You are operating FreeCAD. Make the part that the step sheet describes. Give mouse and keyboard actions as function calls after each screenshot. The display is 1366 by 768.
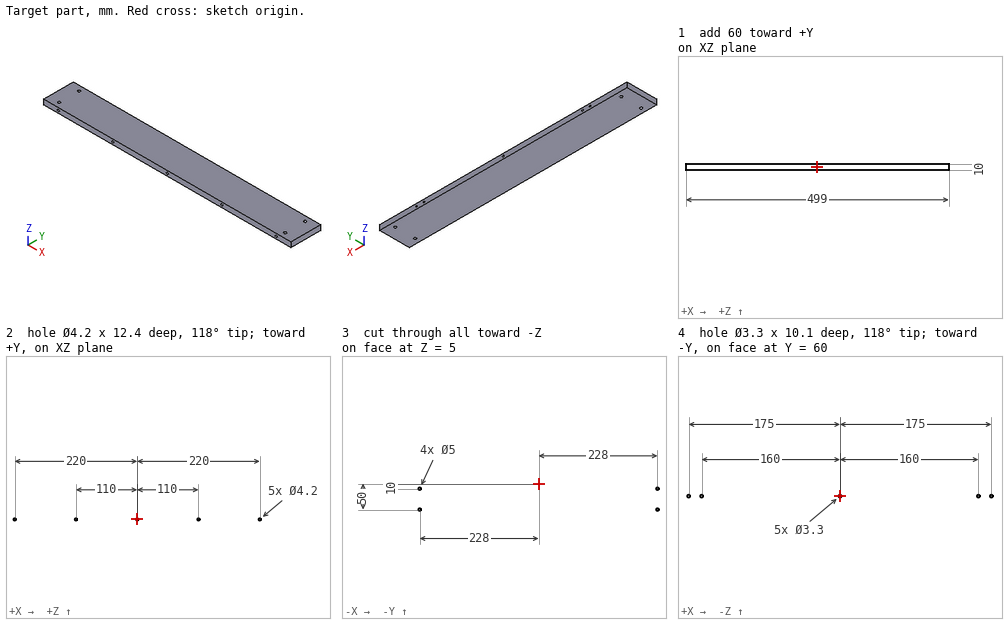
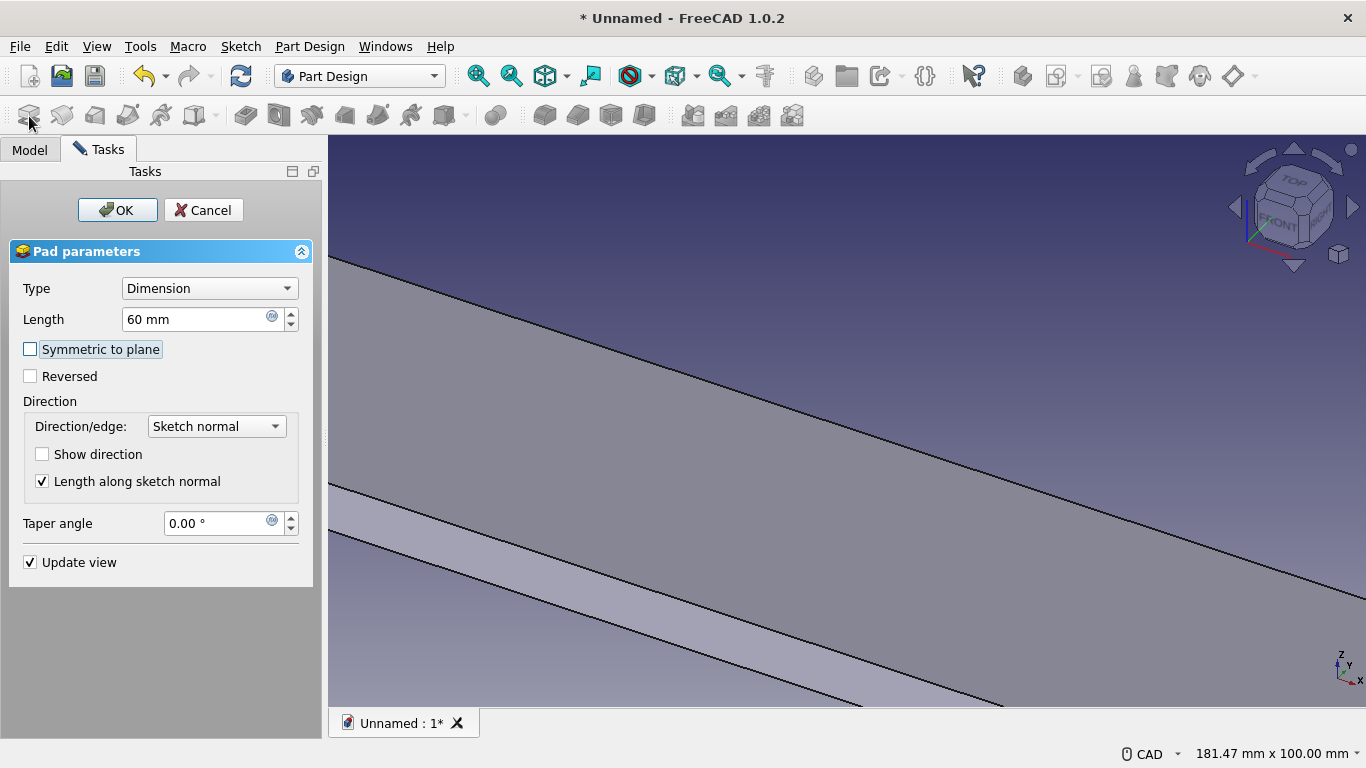
click(31, 376)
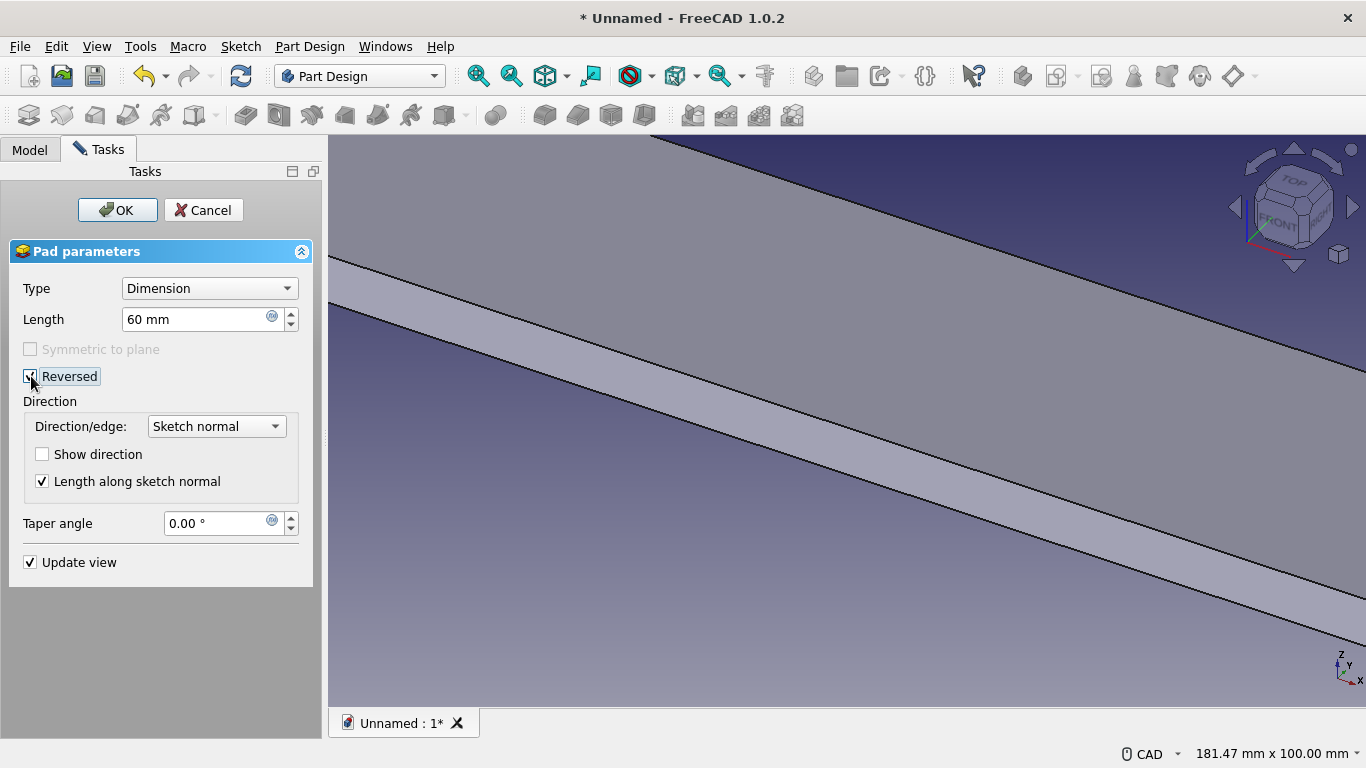
click(118, 210)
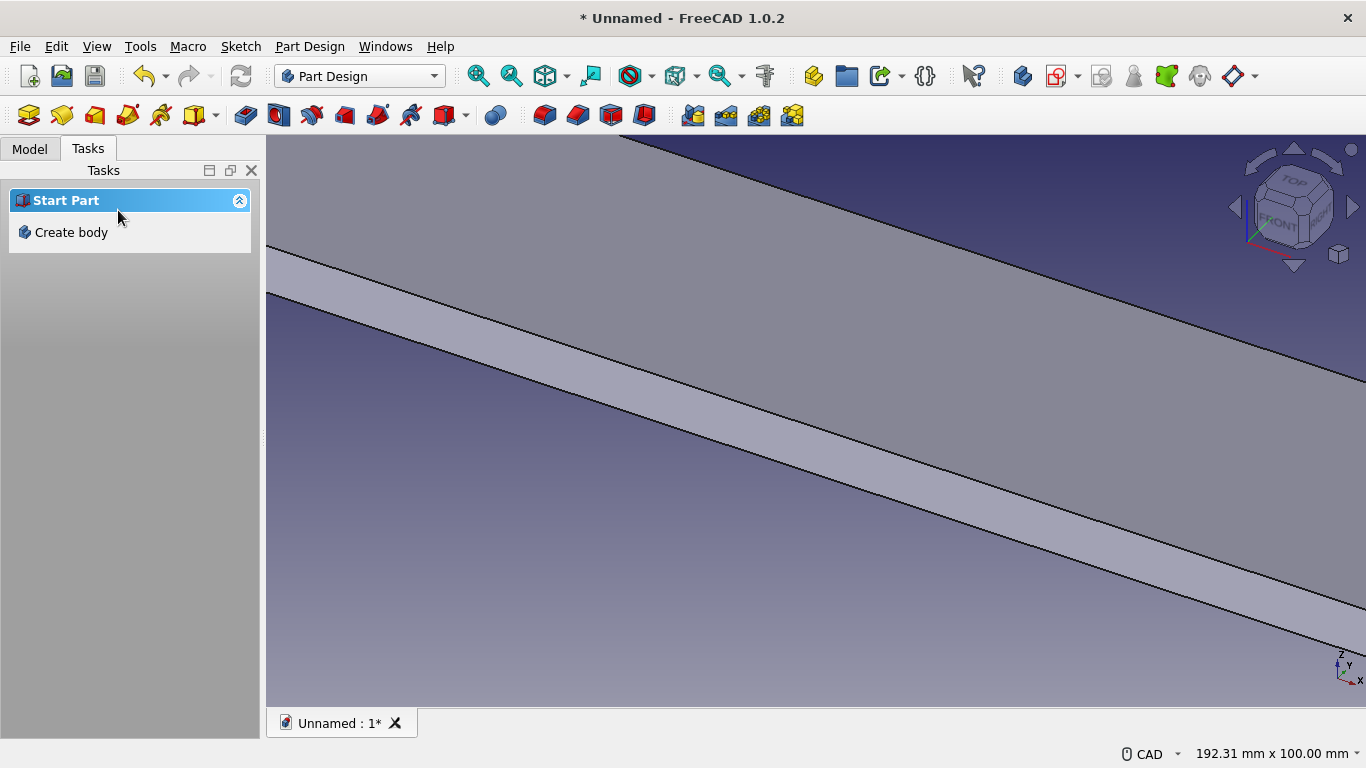
key(v)
key(f)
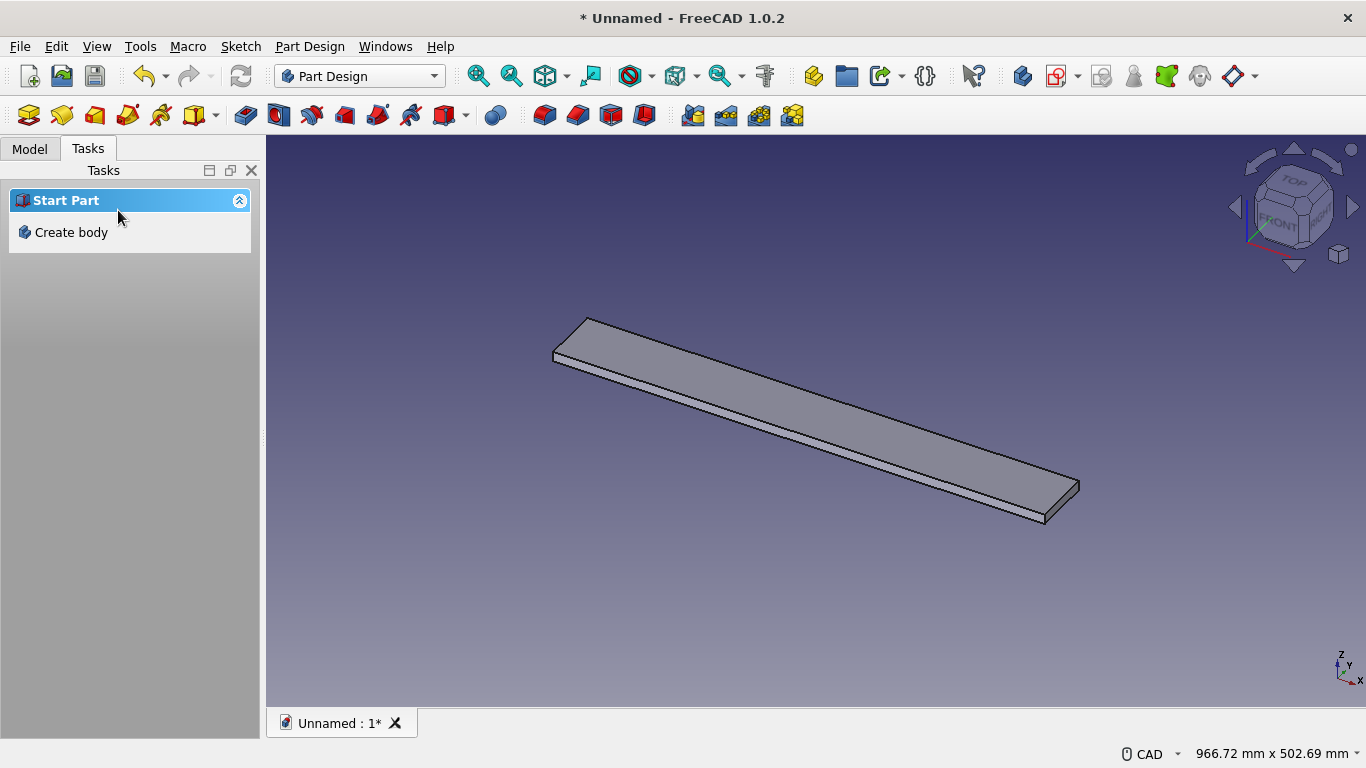
click(1056, 76)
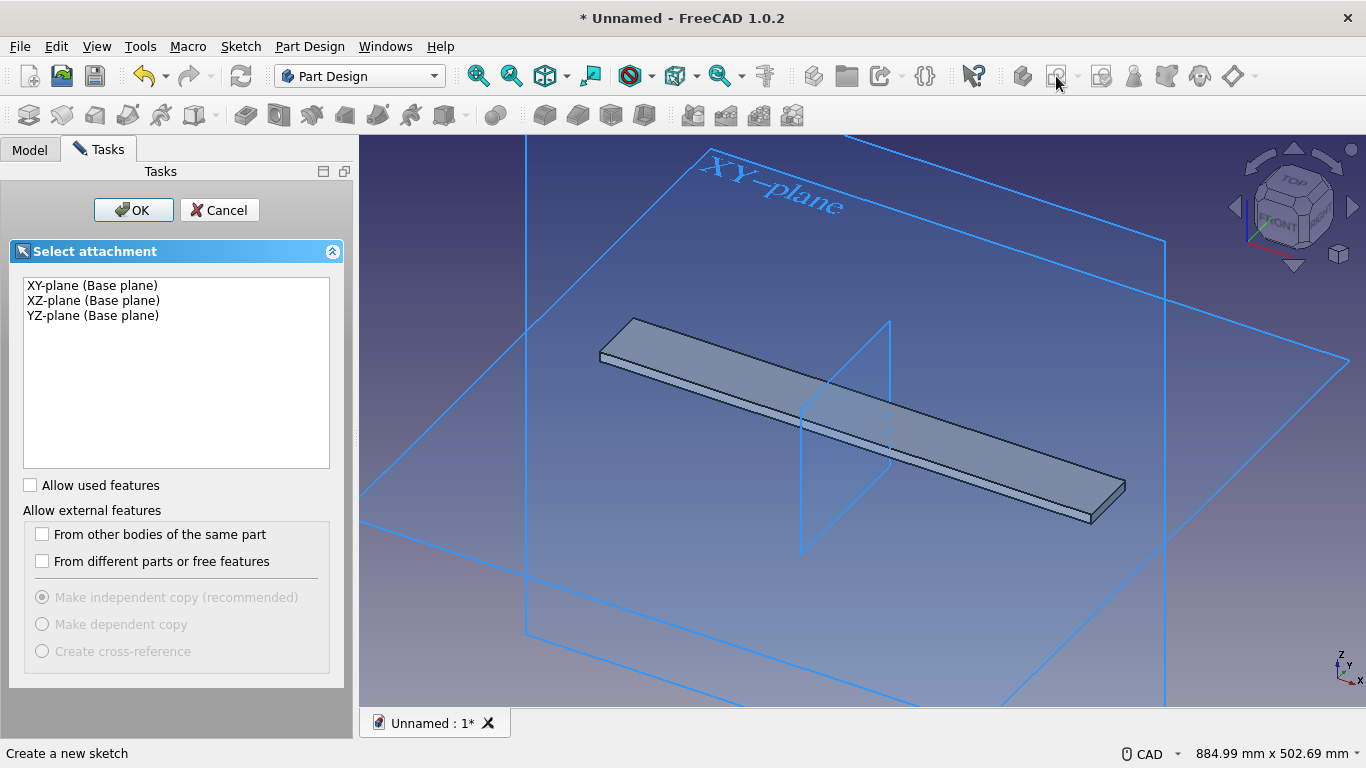
click(84, 300)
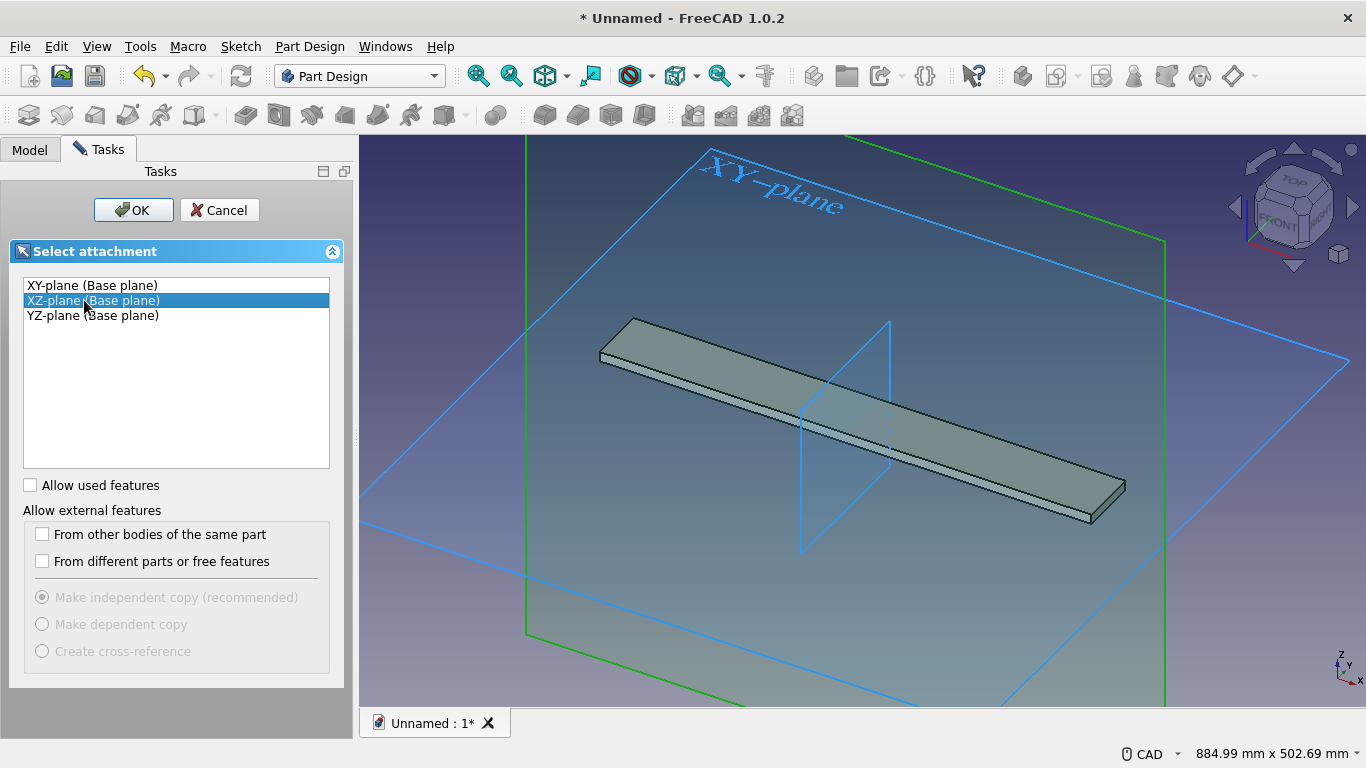
click(134, 210)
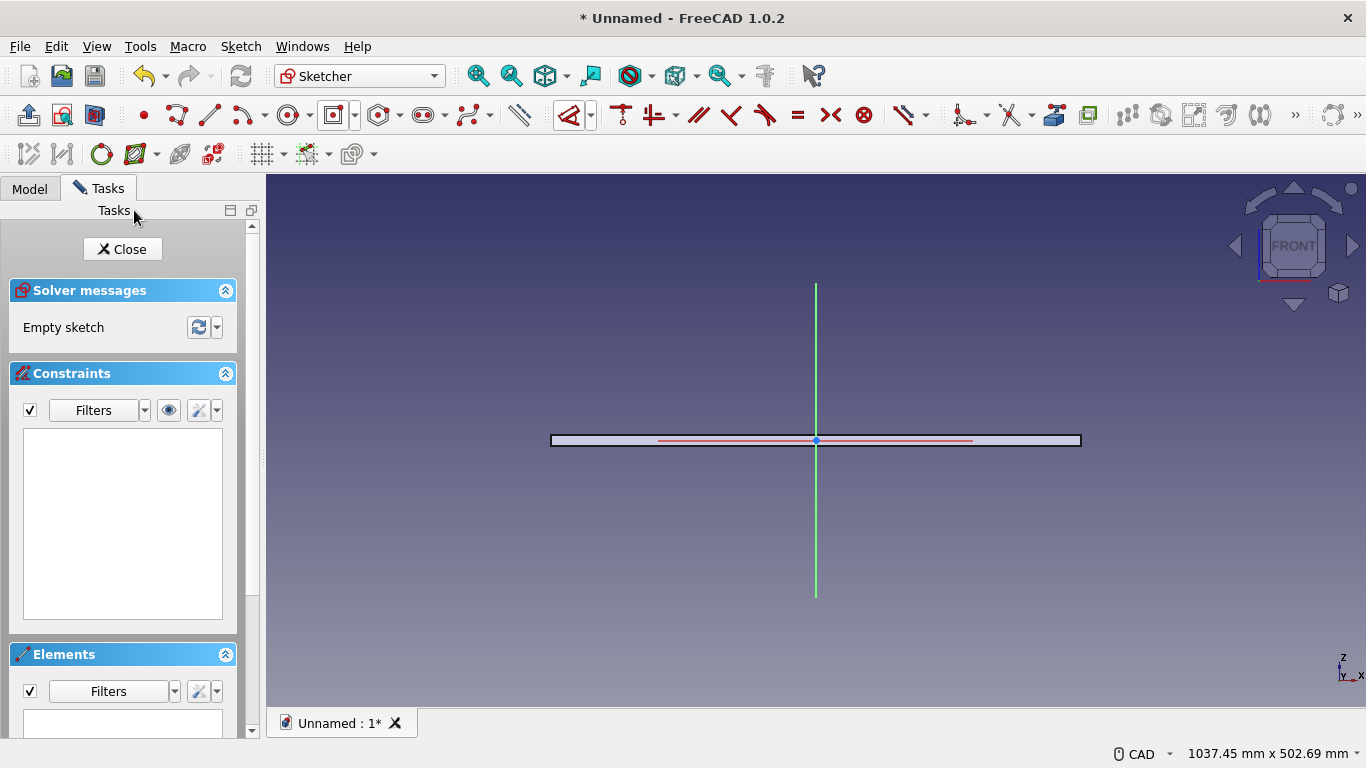
scroll(955, 440, up, 2)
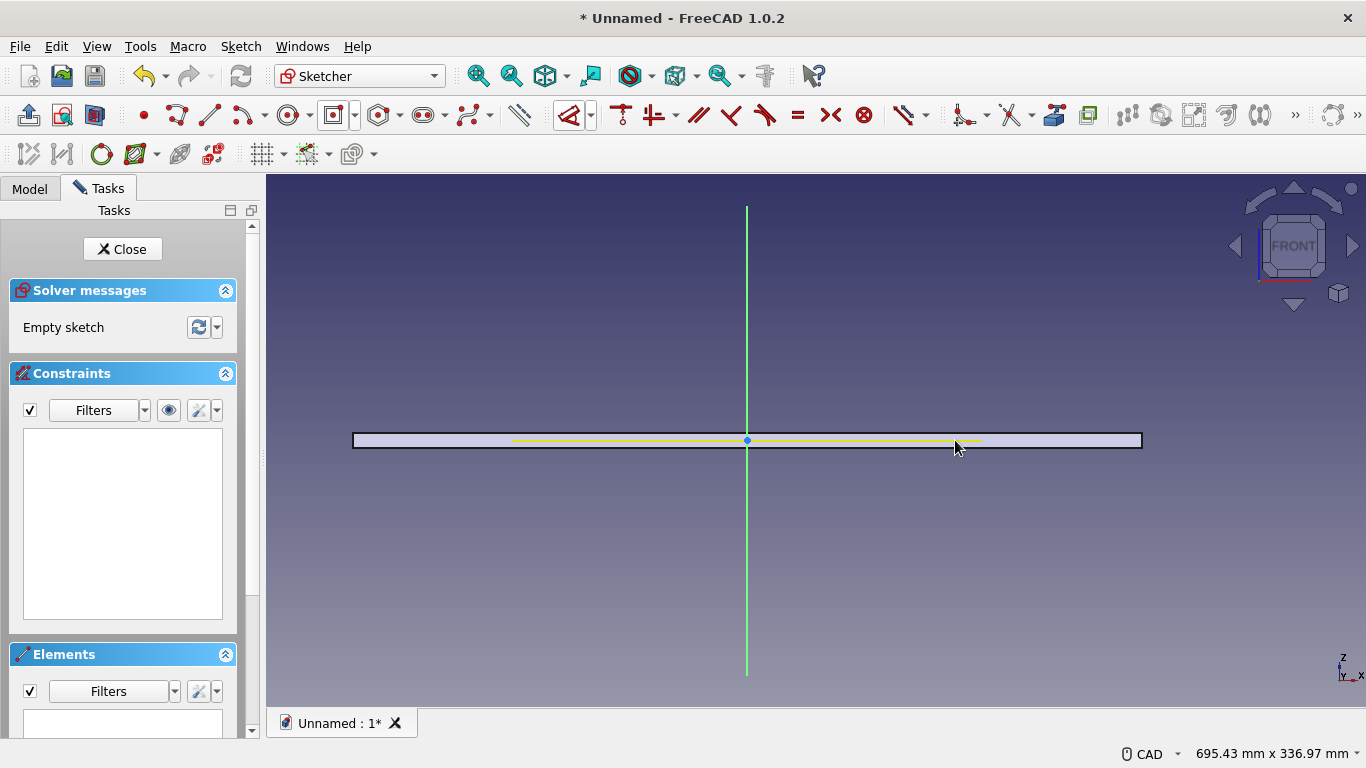
click(288, 116)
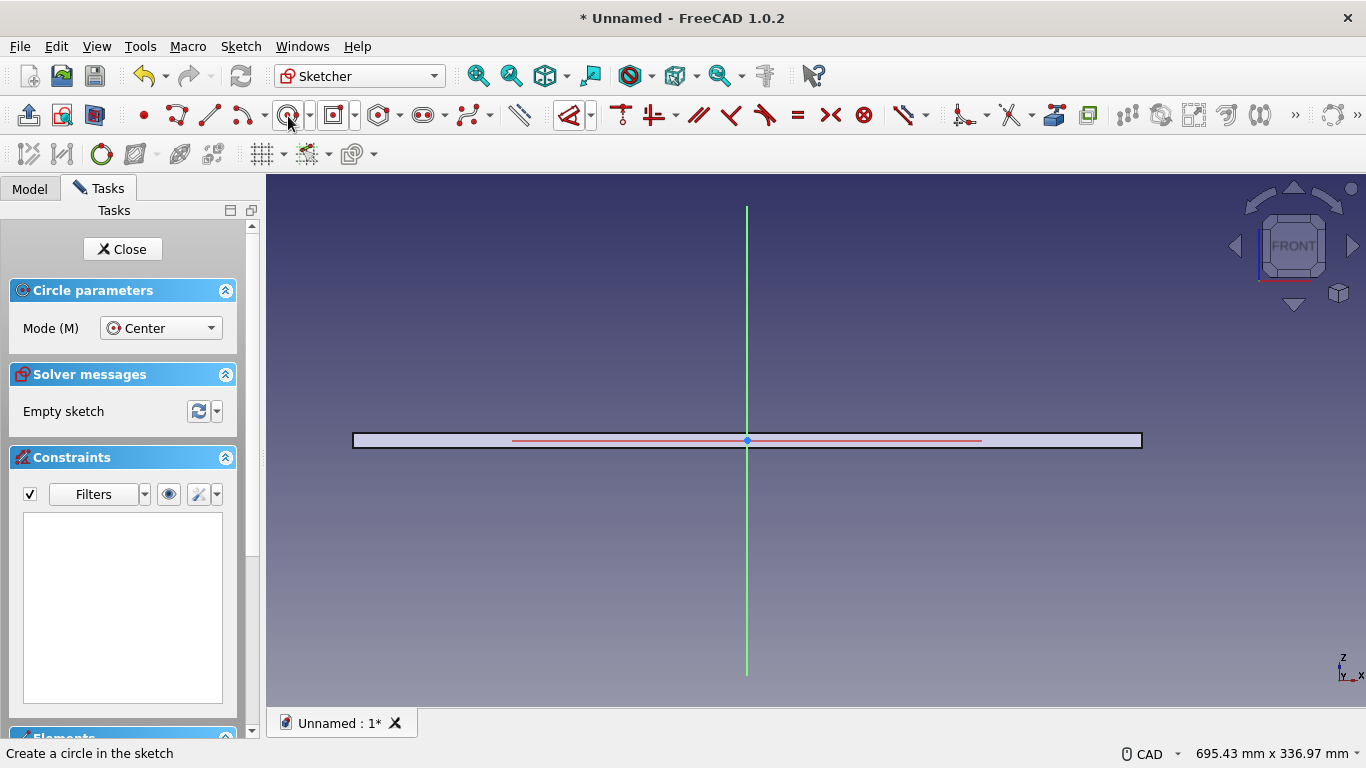
scroll(1095, 440, up, 10)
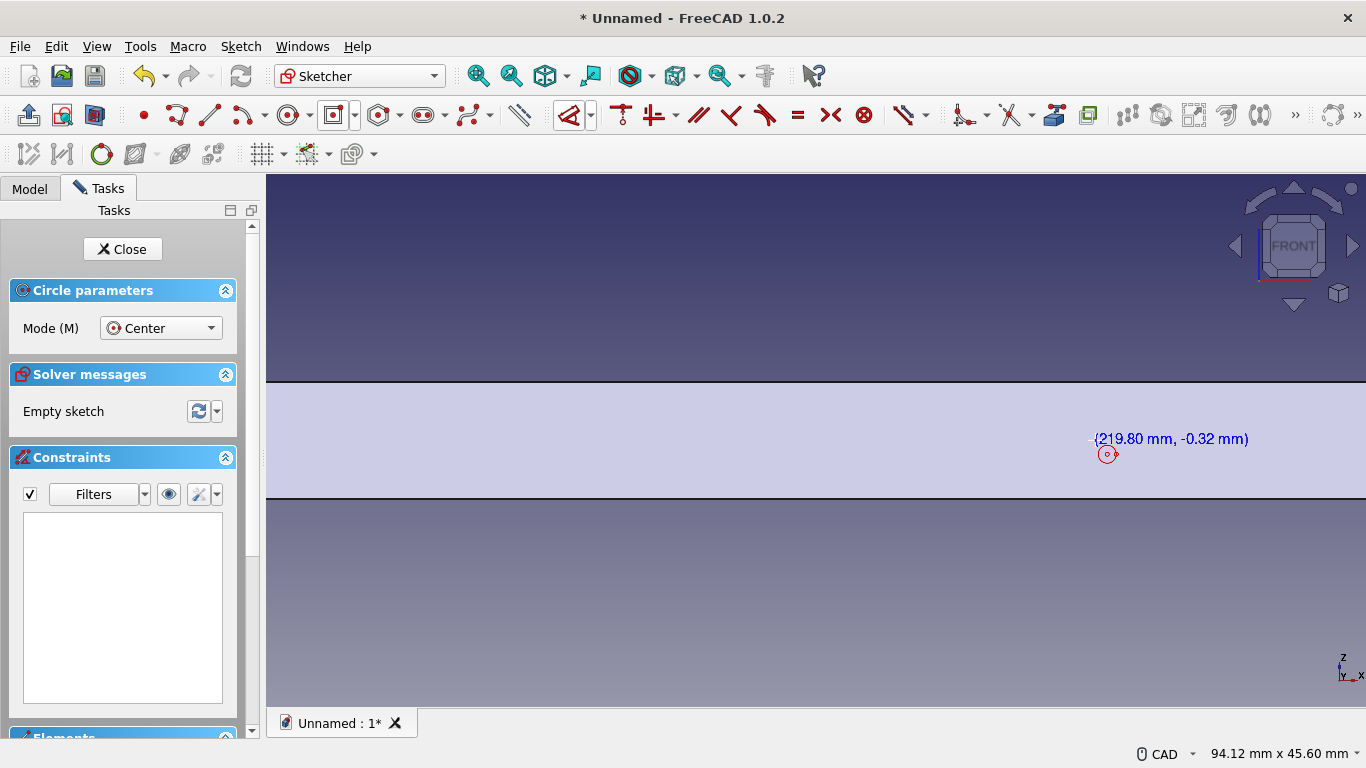
scroll(1096, 440, down, 10)